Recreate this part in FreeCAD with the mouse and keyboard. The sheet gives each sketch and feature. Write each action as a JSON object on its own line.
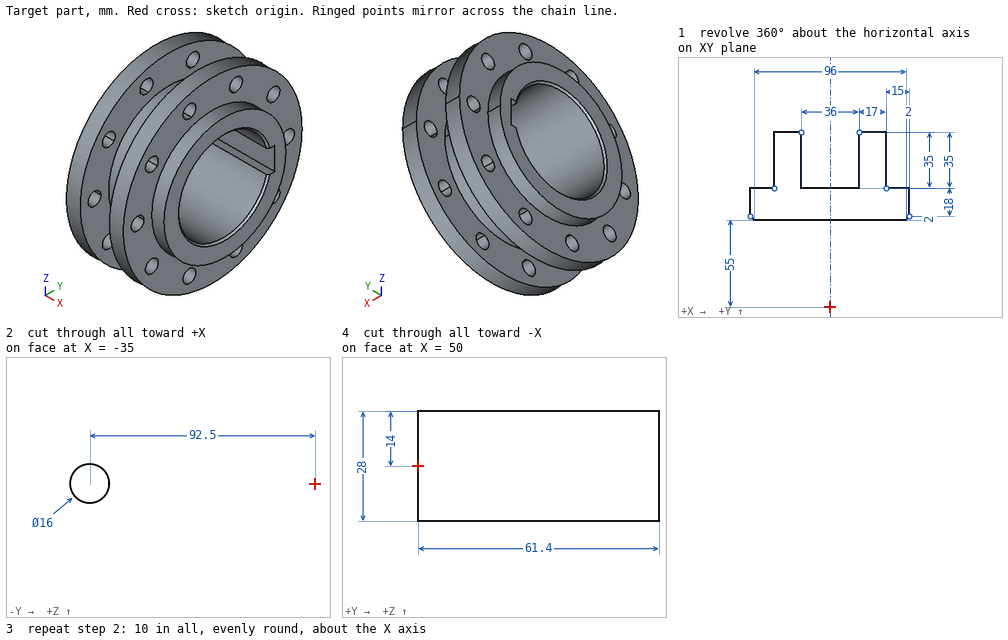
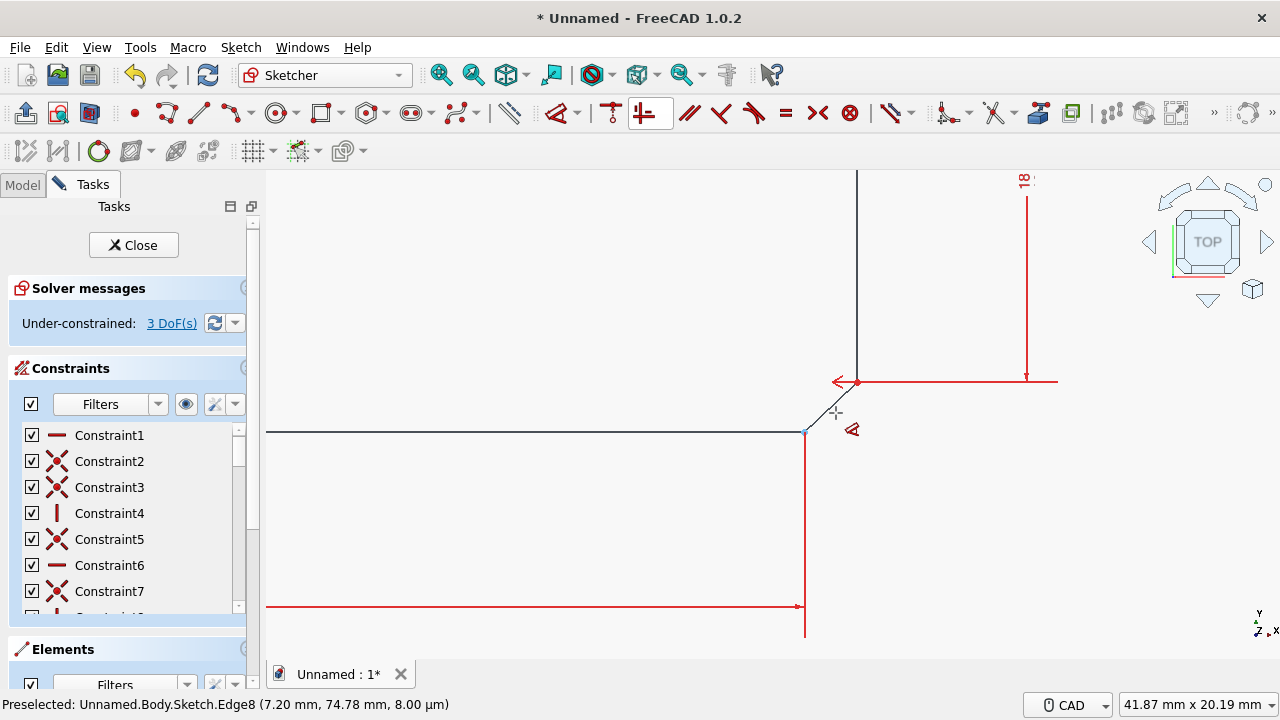
{"action": "left_click", "coordinate": [831, 407]}
{"action": "left_click", "coordinate": [831, 348]}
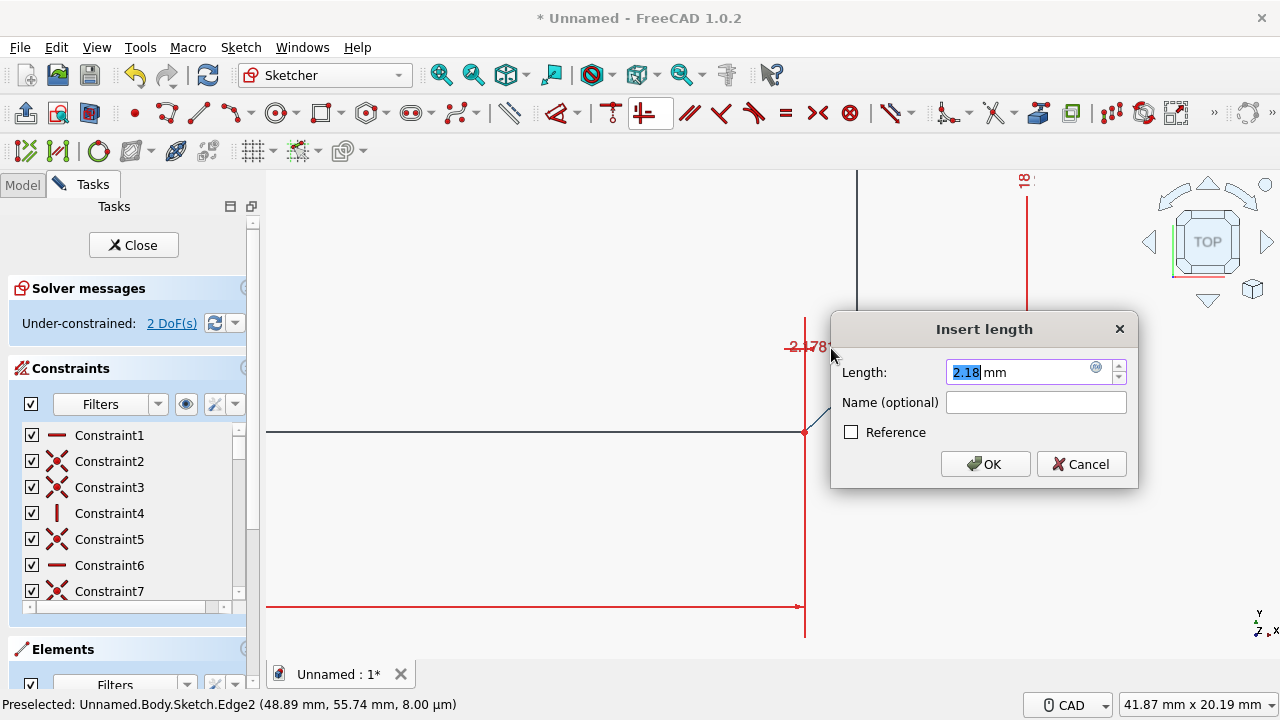
{"action": "type", "text": "2"}
{"action": "key", "text": "Return"}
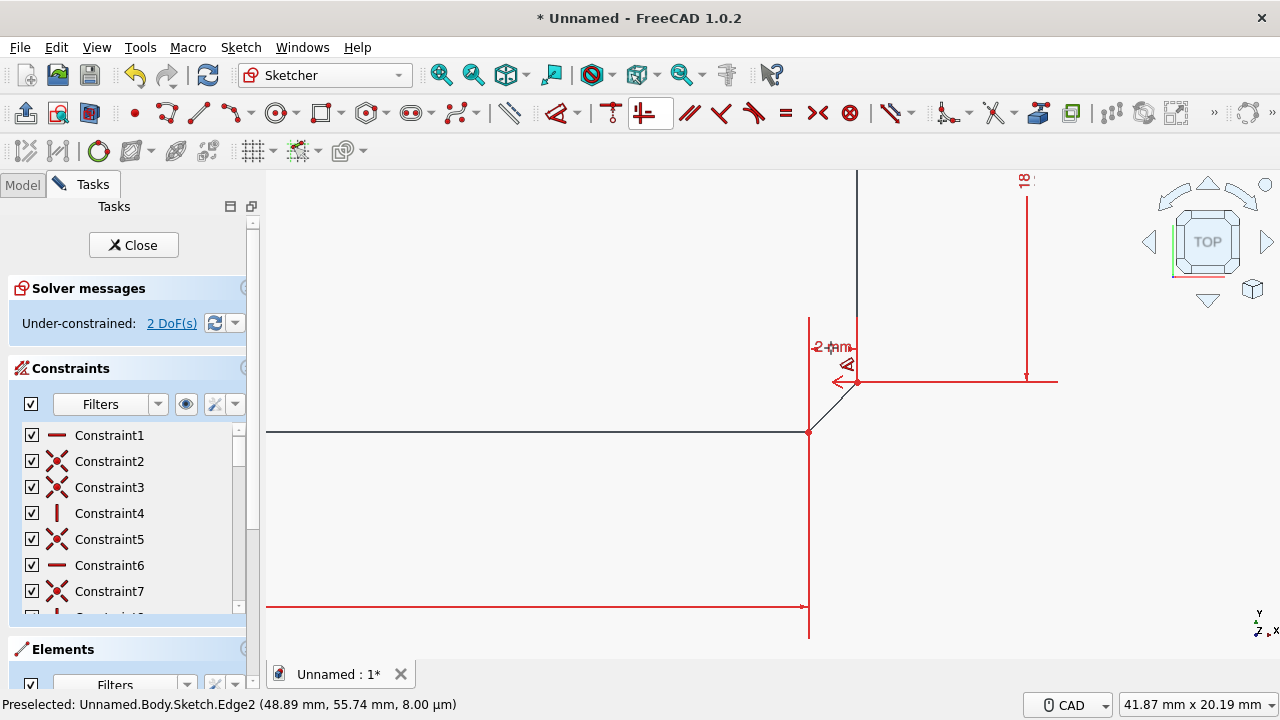
{"action": "left_click", "coordinate": [823, 417]}
{"action": "left_click", "coordinate": [891, 407]}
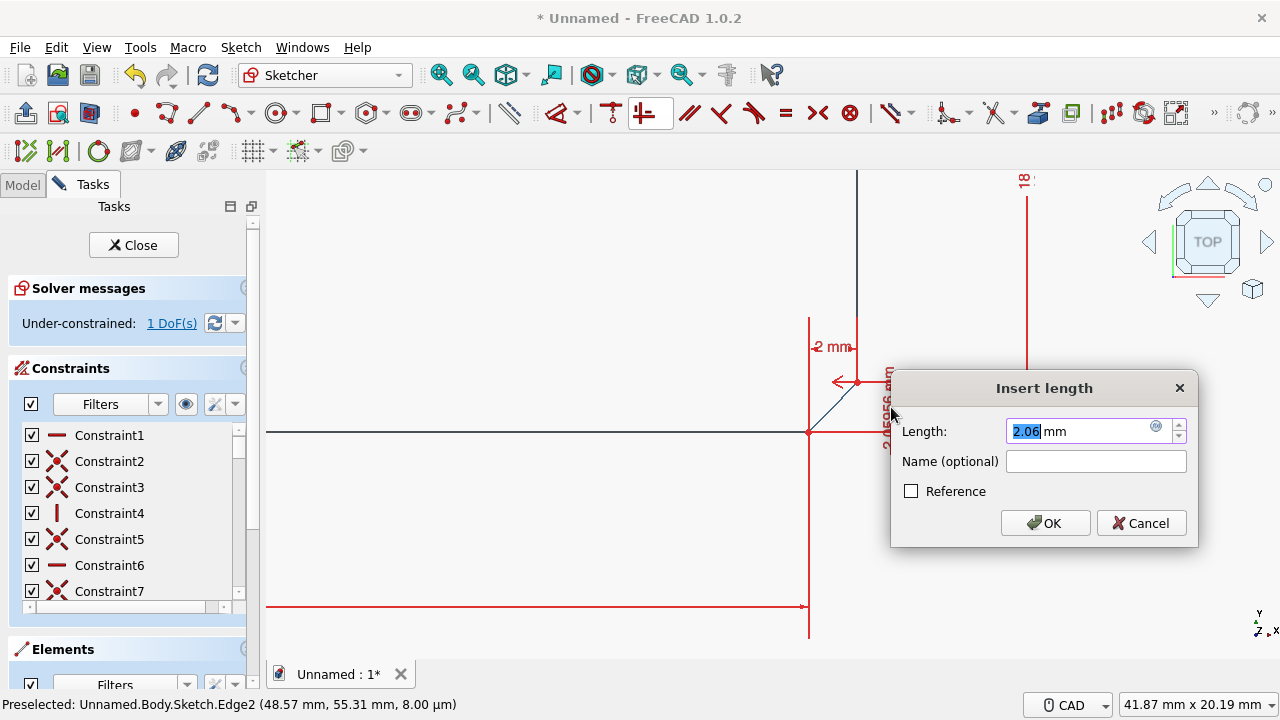
{"action": "type", "text": "2"}
{"action": "key", "text": "Return"}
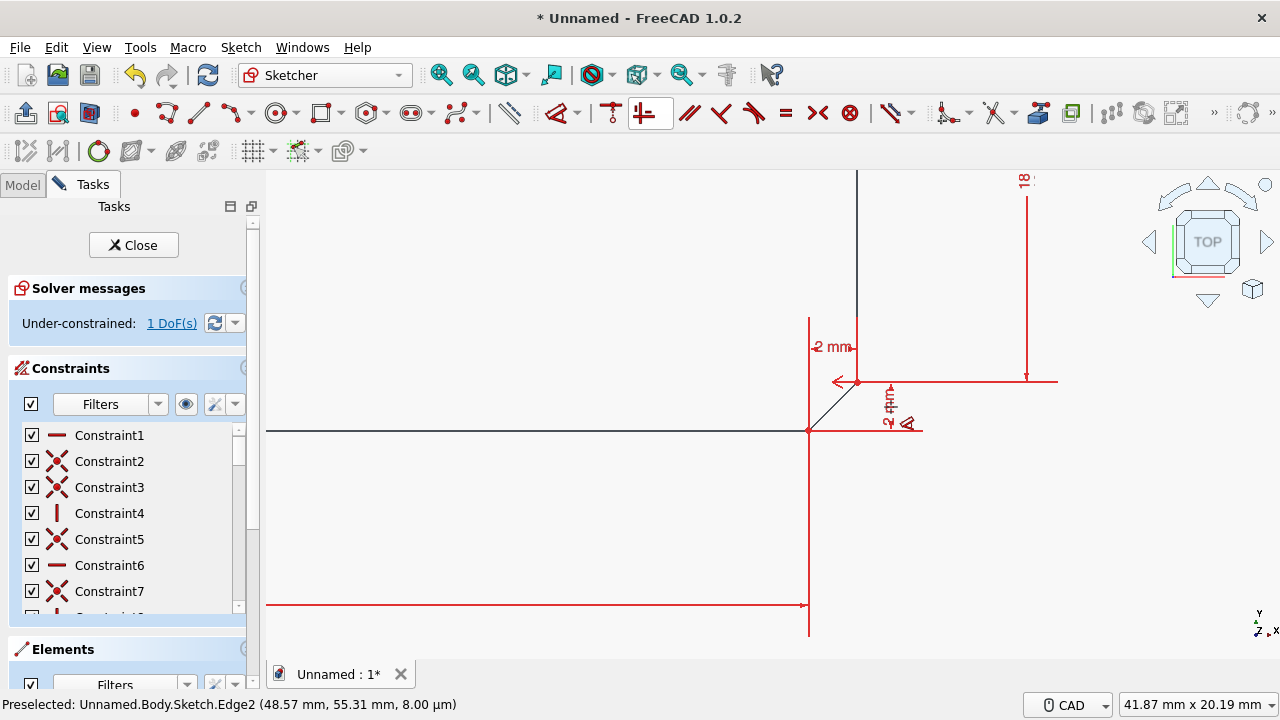
{"action": "scroll", "coordinate": [836, 413], "scroll_direction": "down", "scroll_amount": 11}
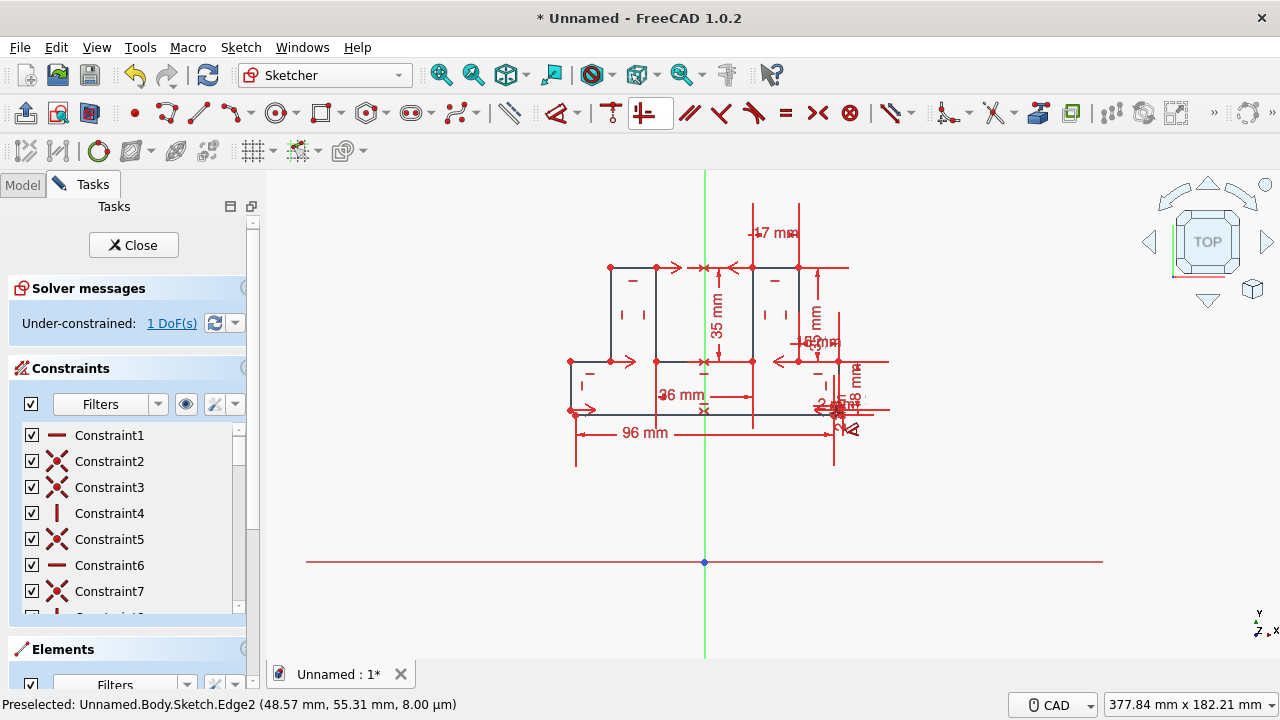
{"action": "scroll", "coordinate": [576, 415], "scroll_direction": "up", "scroll_amount": 3}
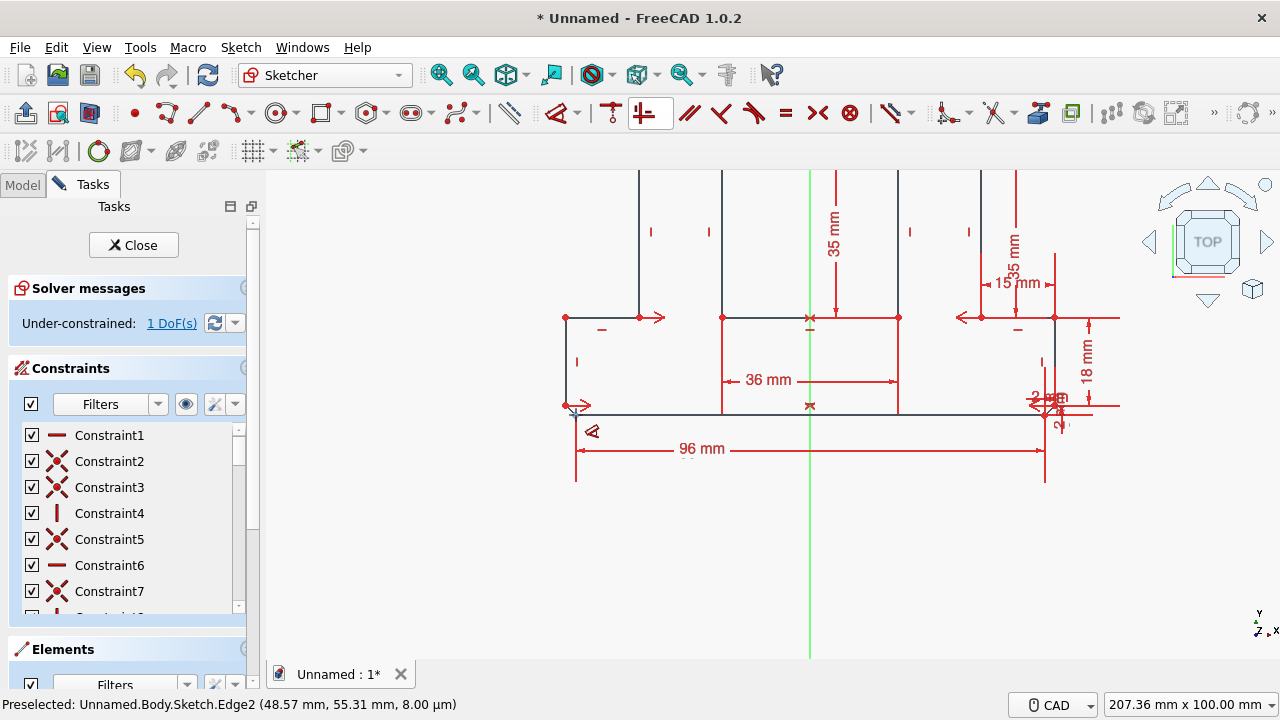
{"action": "left_click", "coordinate": [576, 415]}
{"action": "left_click", "coordinate": [542, 523]}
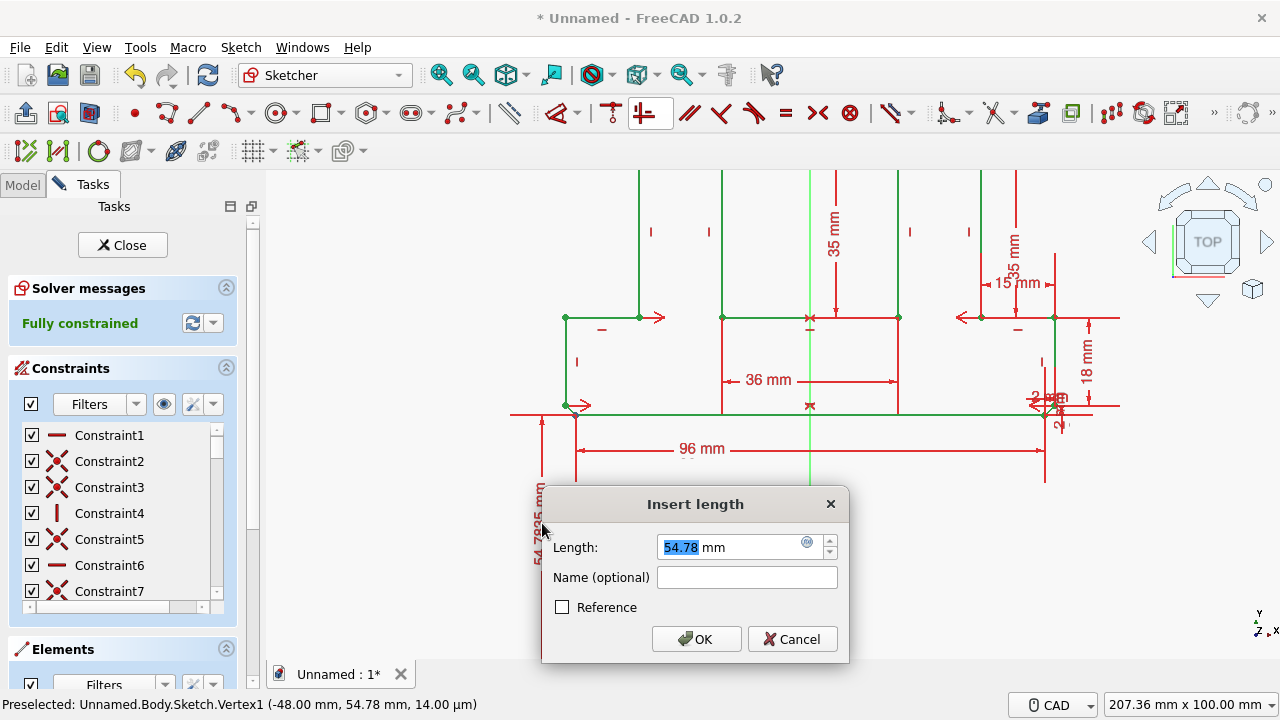
{"action": "type", "text": "55"}
{"action": "key", "text": "Return"}
{"action": "key", "text": "Escape"}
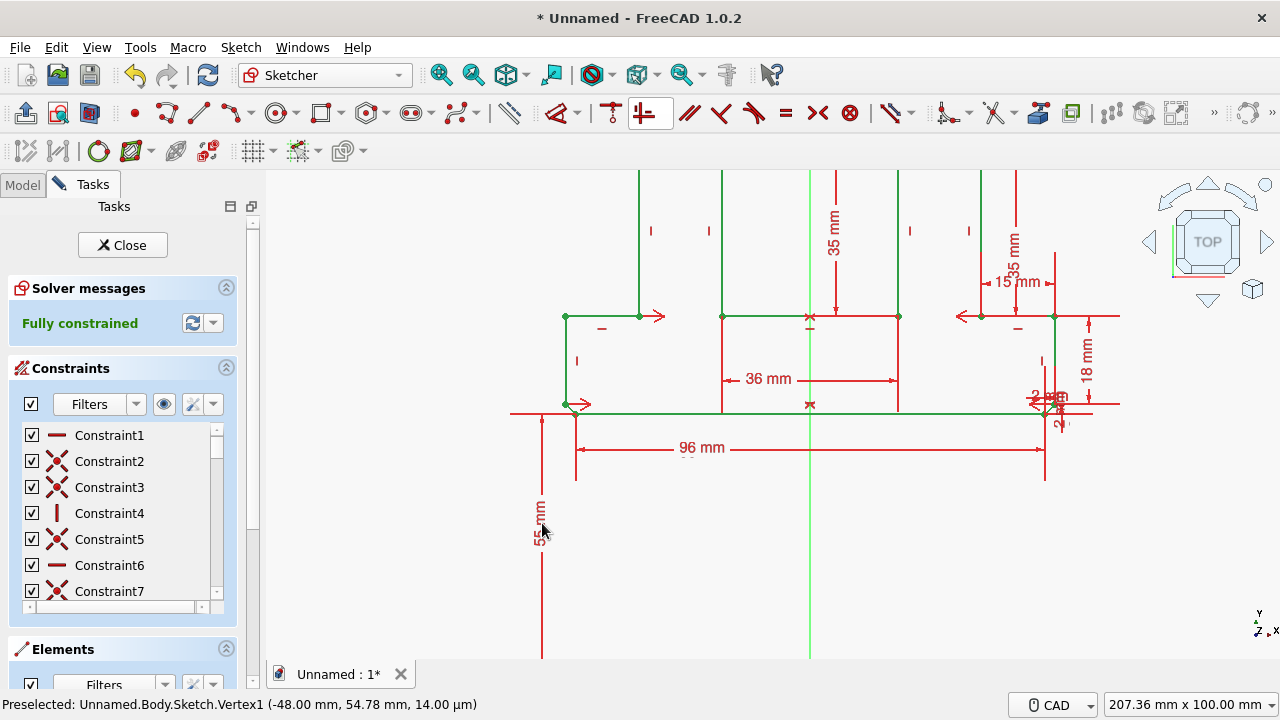
{"action": "left_click", "coordinate": [123, 245]}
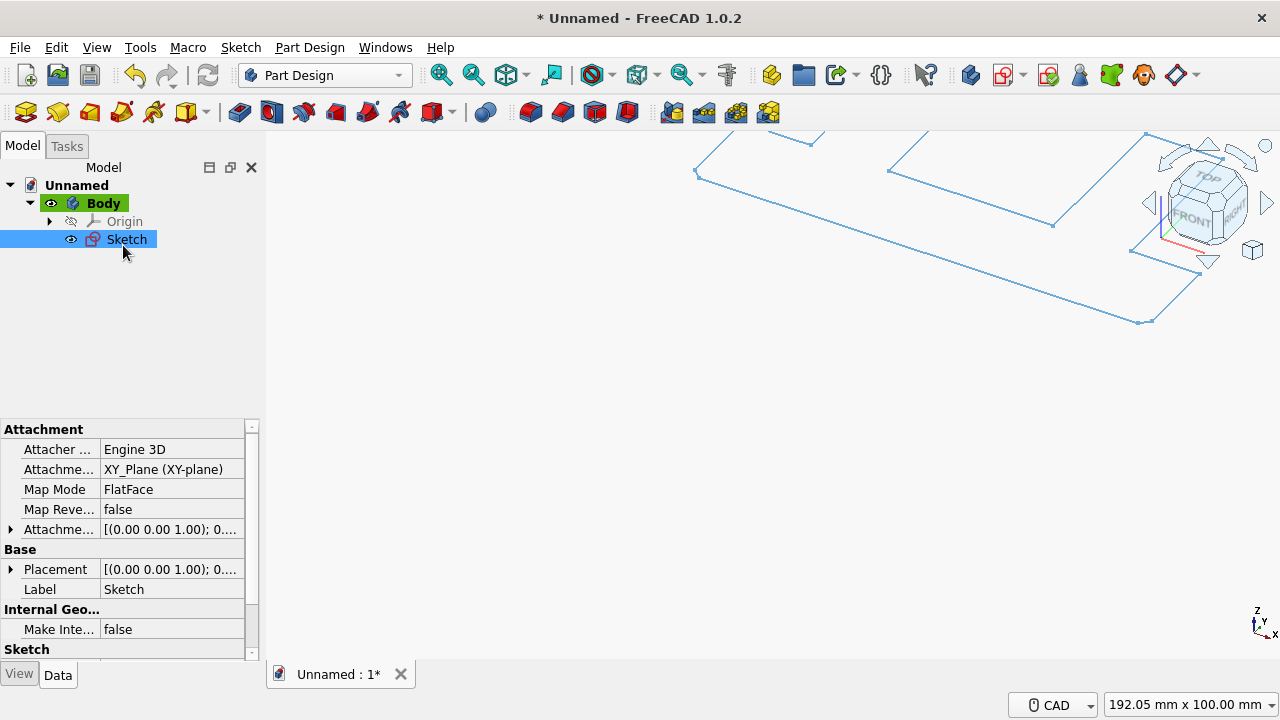
{"action": "left_click", "coordinate": [58, 112]}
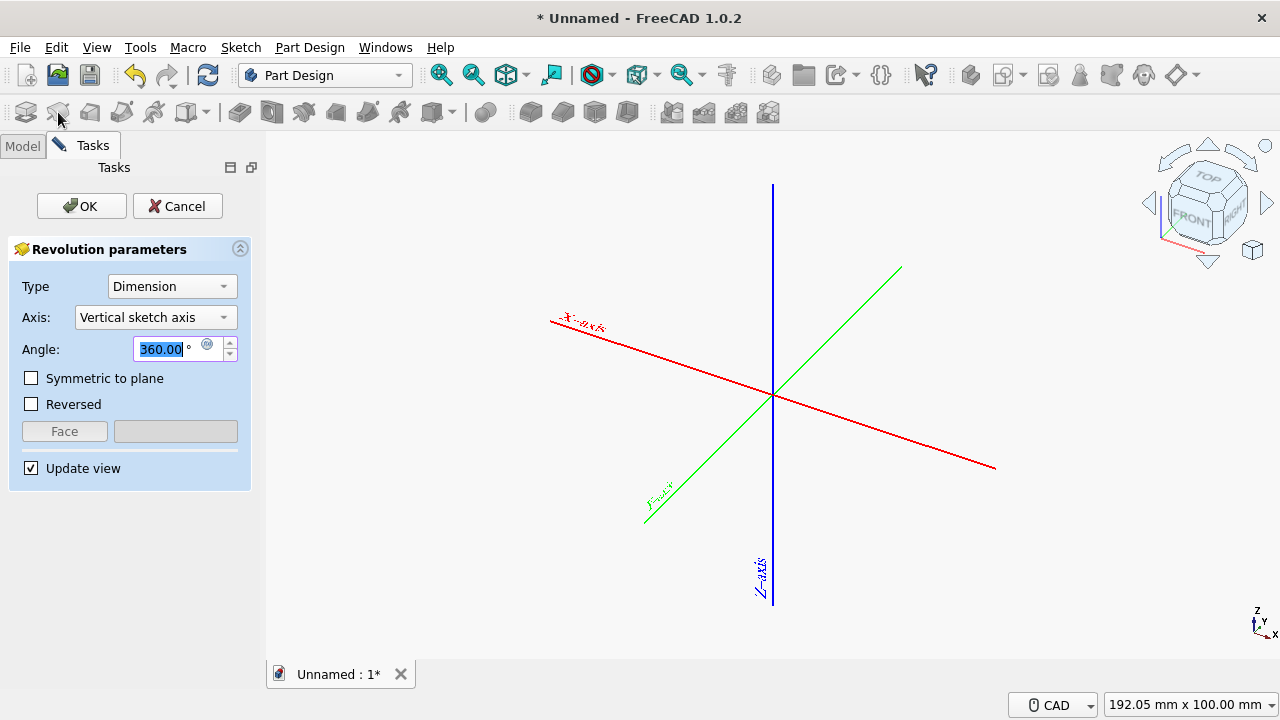
{"action": "left_click", "coordinate": [156, 318]}